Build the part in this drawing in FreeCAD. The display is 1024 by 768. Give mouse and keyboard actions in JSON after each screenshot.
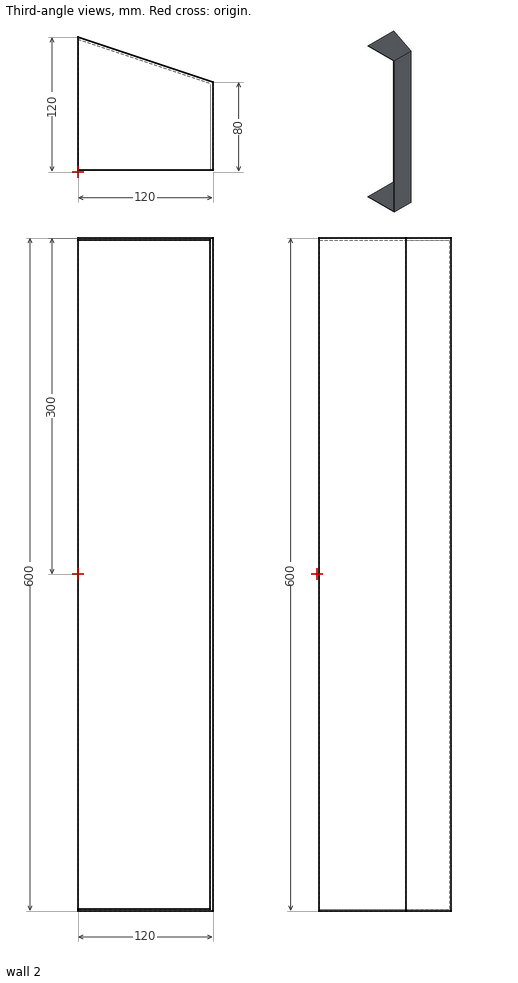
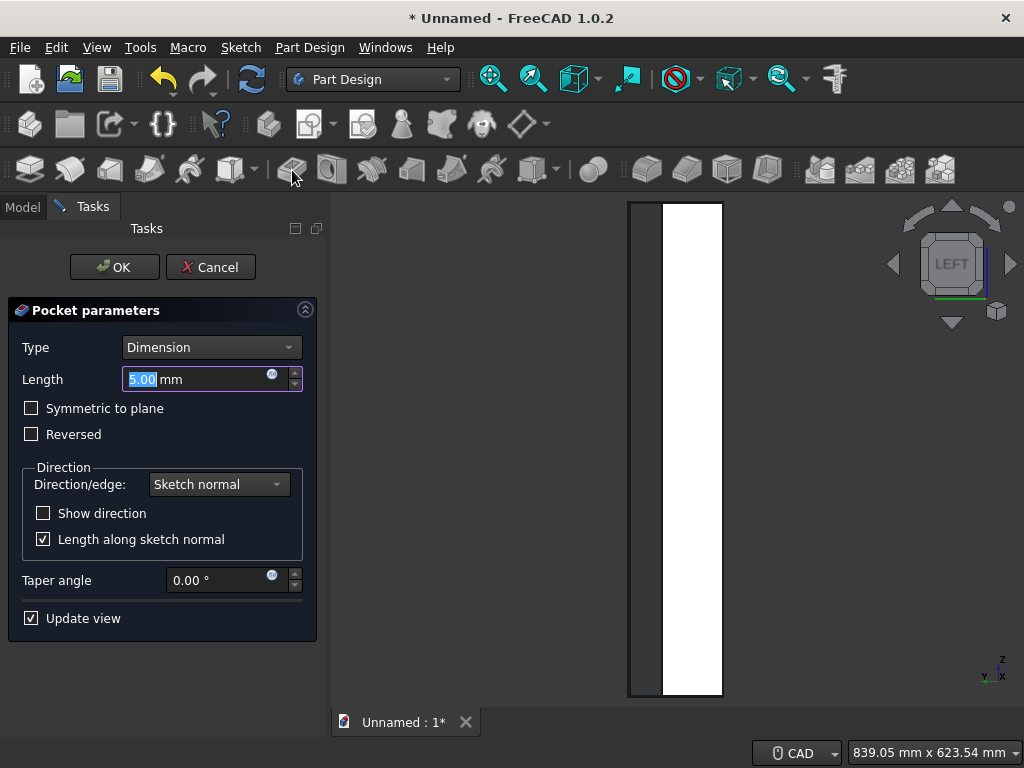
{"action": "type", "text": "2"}
{"action": "key", "text": "Tab"}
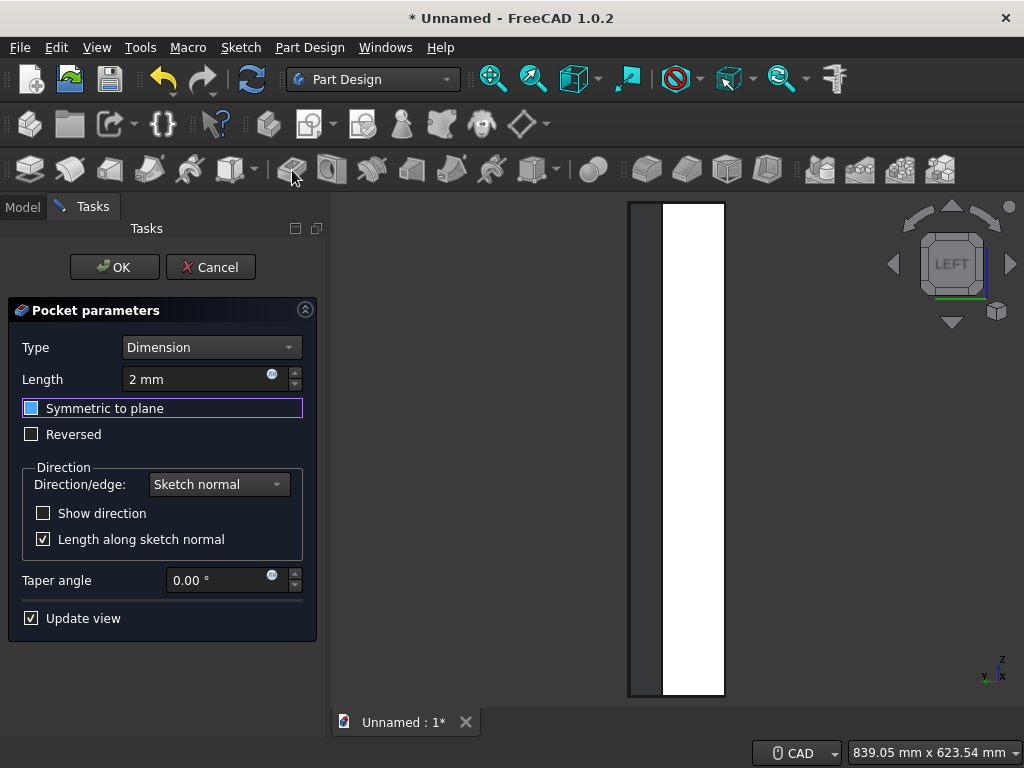
{"action": "left_click", "coordinate": [115, 267]}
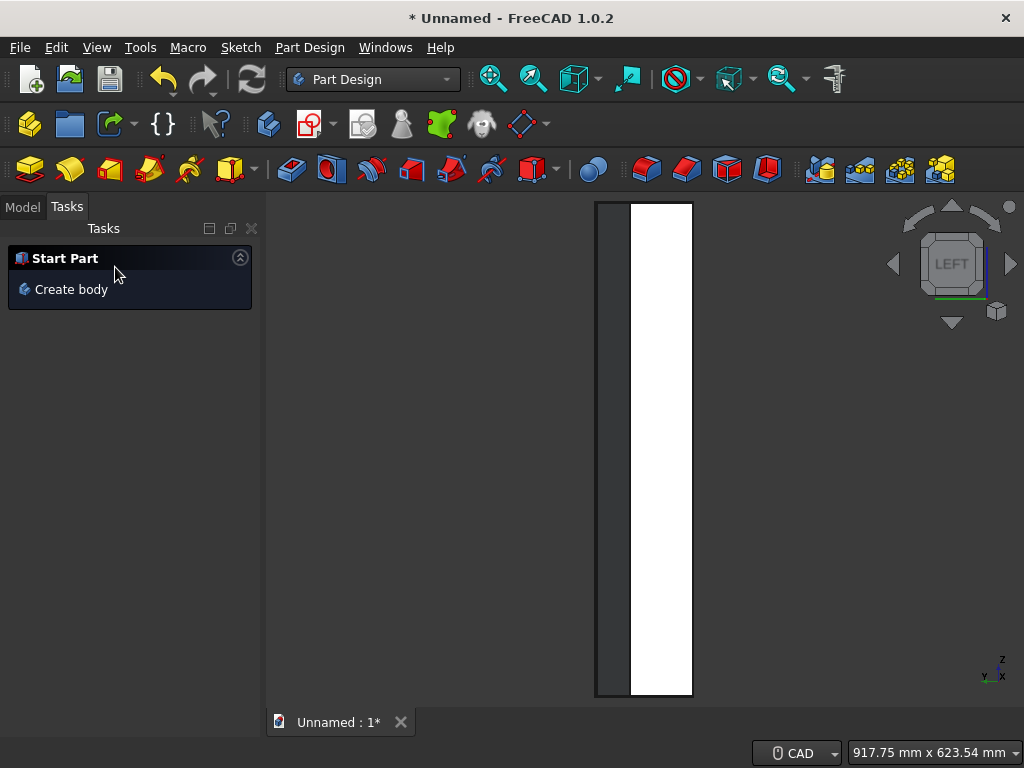
{"action": "key", "text": "0"}